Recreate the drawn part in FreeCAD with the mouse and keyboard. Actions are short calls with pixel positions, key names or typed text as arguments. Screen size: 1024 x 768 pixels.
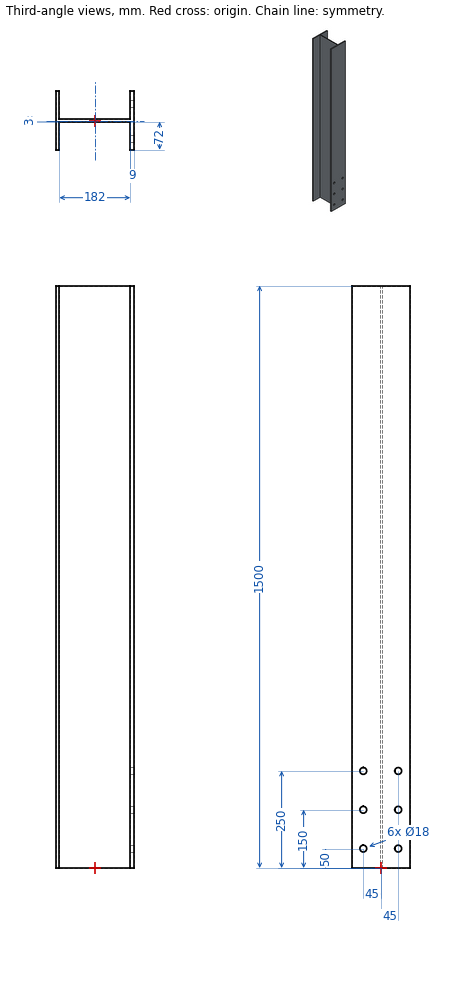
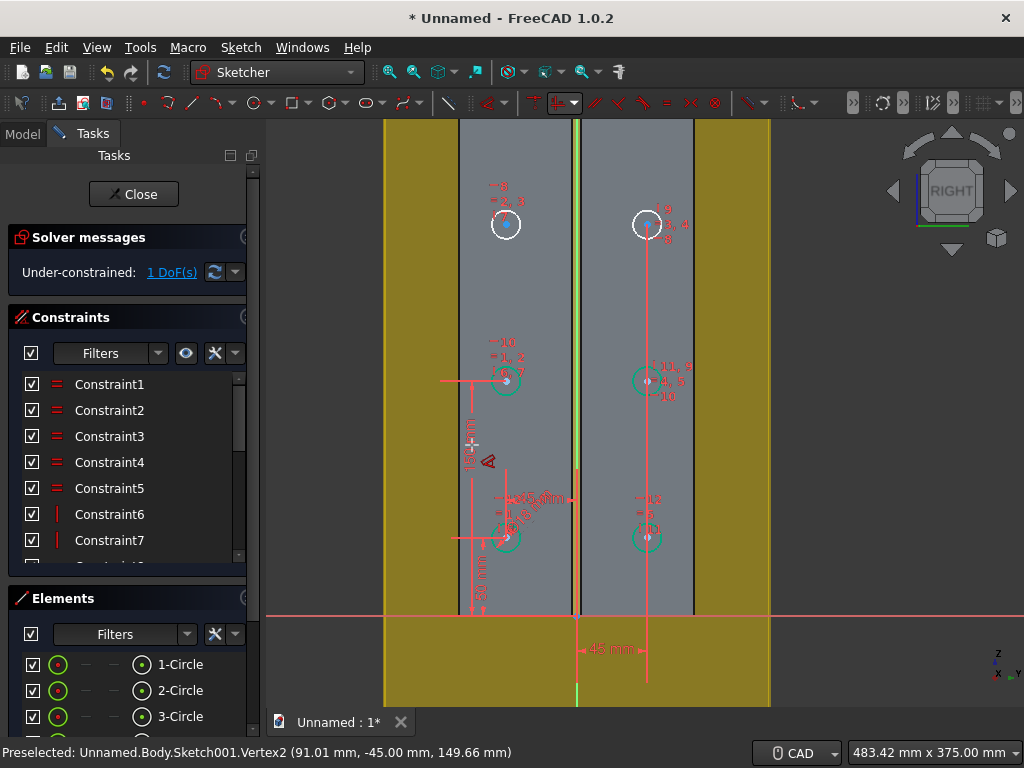
click(506, 225)
click(472, 420)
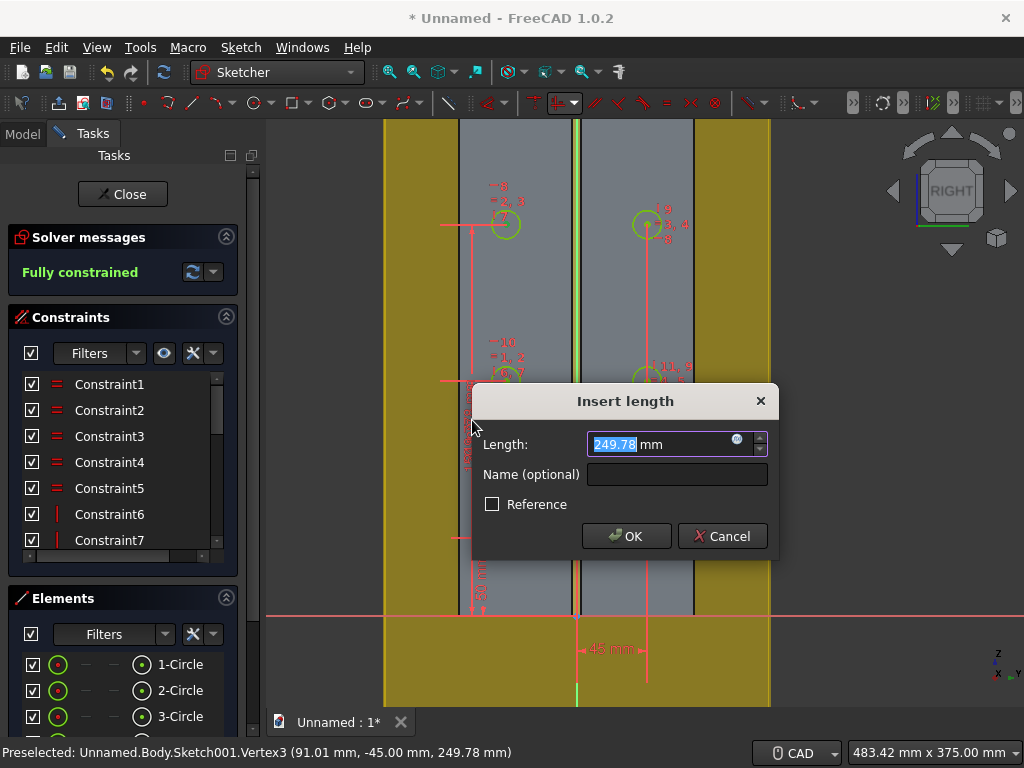
text(250)
key(Return)
key(Escape)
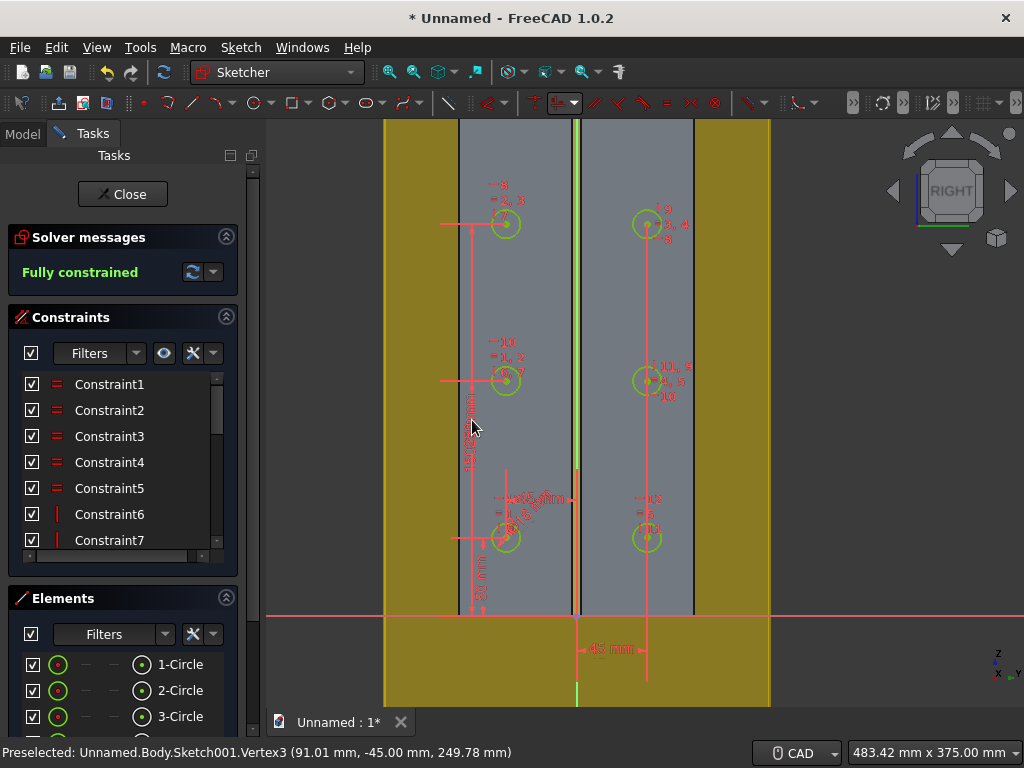
click(123, 194)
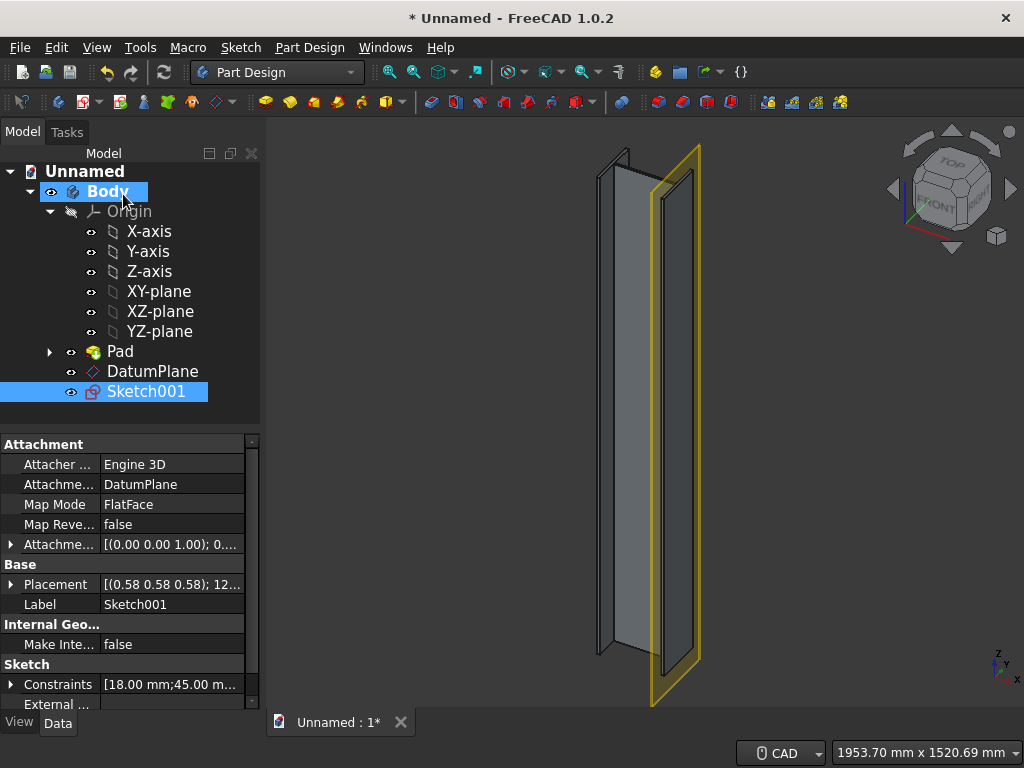
click(432, 102)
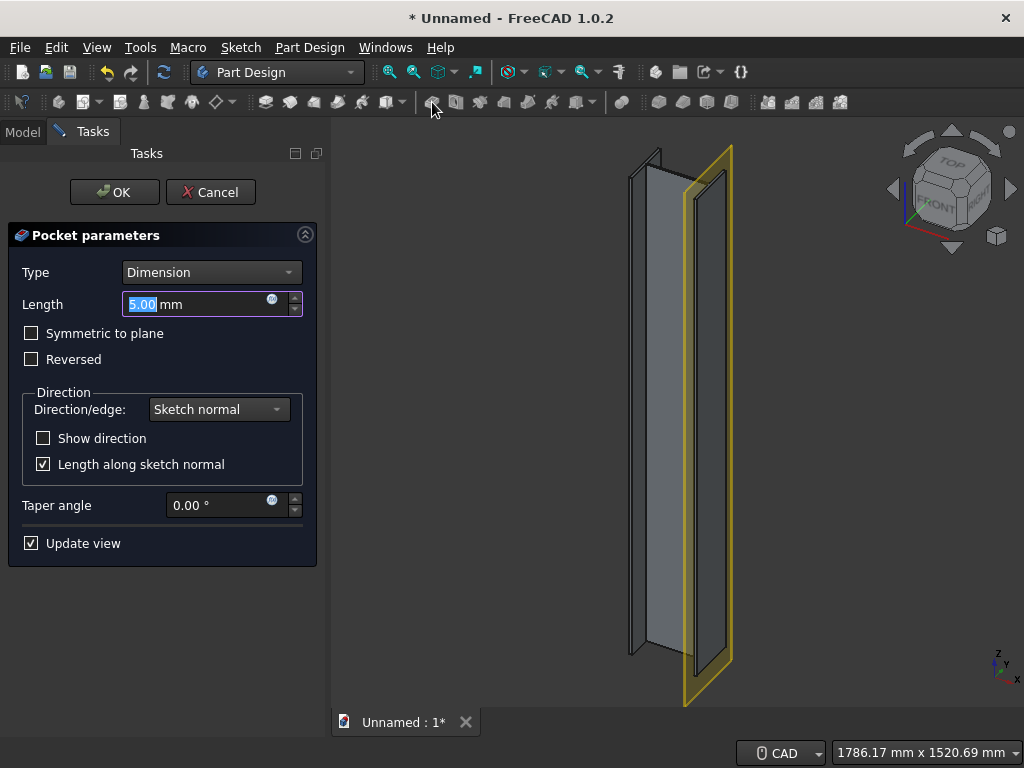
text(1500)
key(Tab)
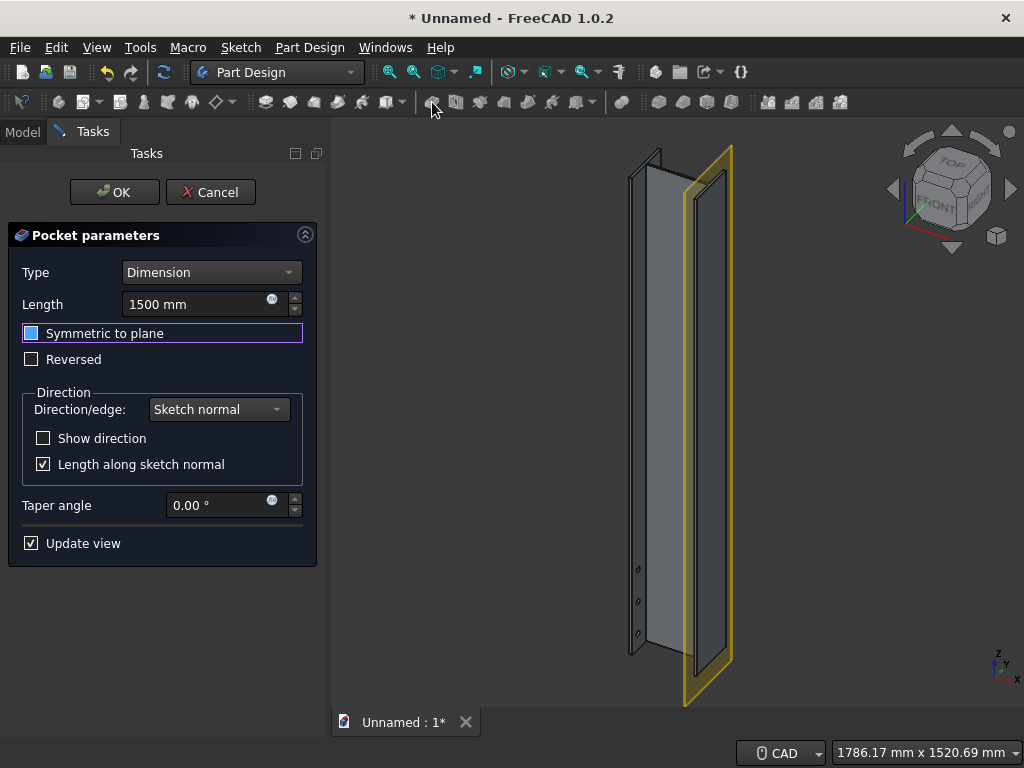
click(30, 359)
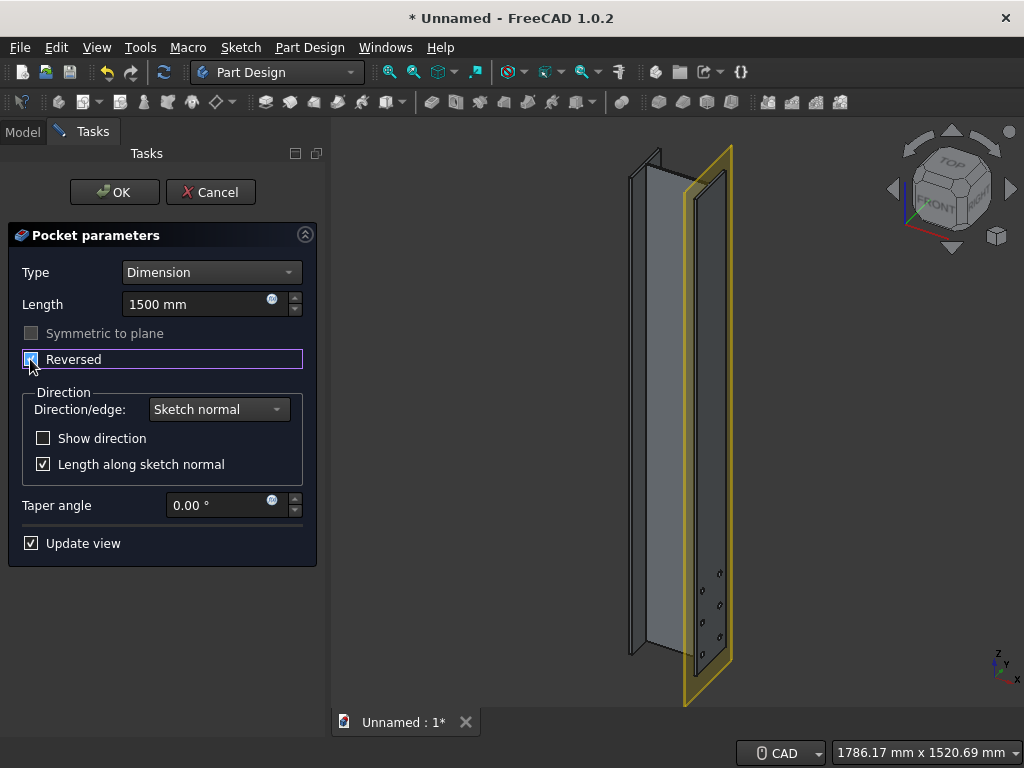
click(115, 192)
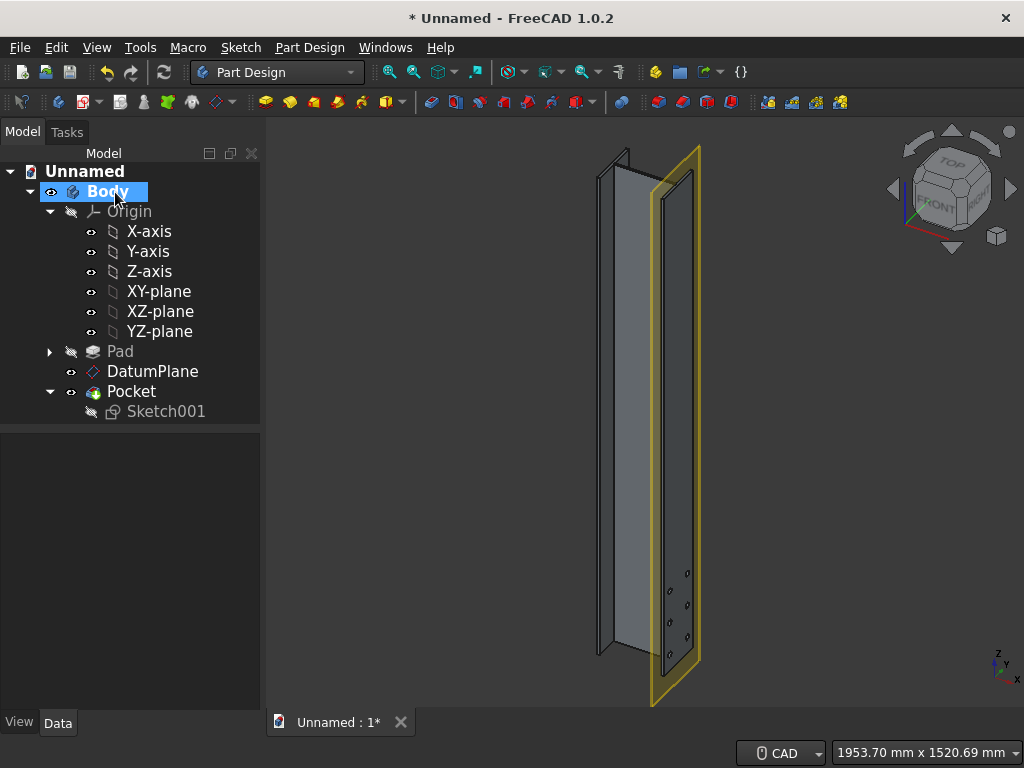
click(116, 372)
key(space)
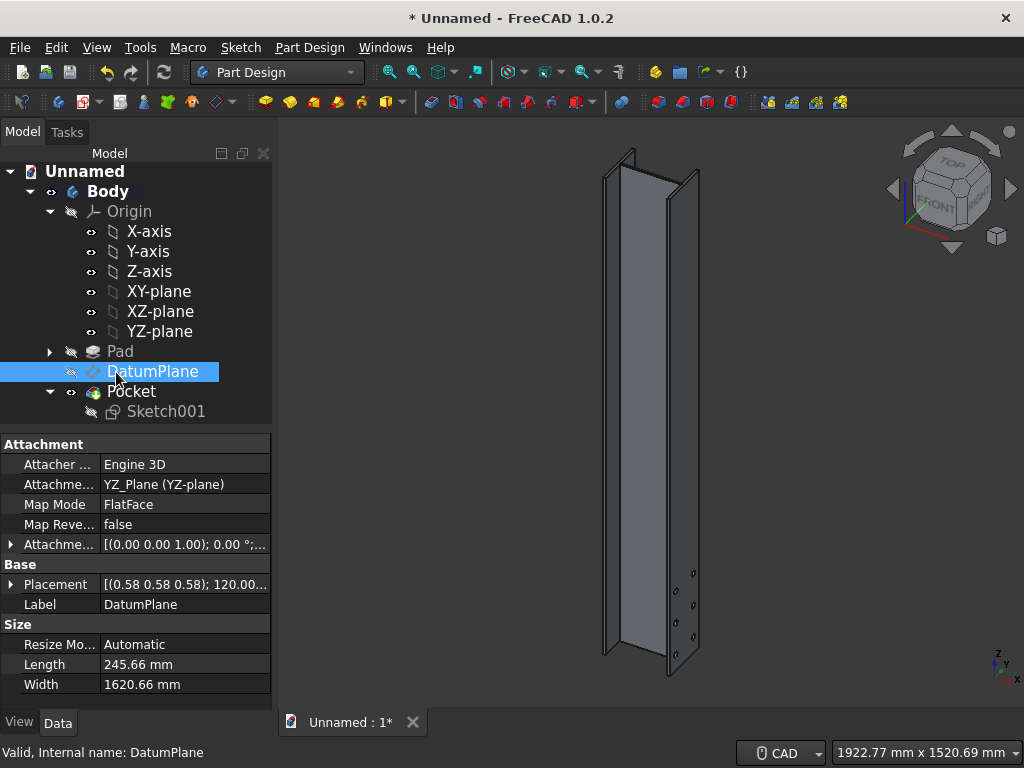
key(0)